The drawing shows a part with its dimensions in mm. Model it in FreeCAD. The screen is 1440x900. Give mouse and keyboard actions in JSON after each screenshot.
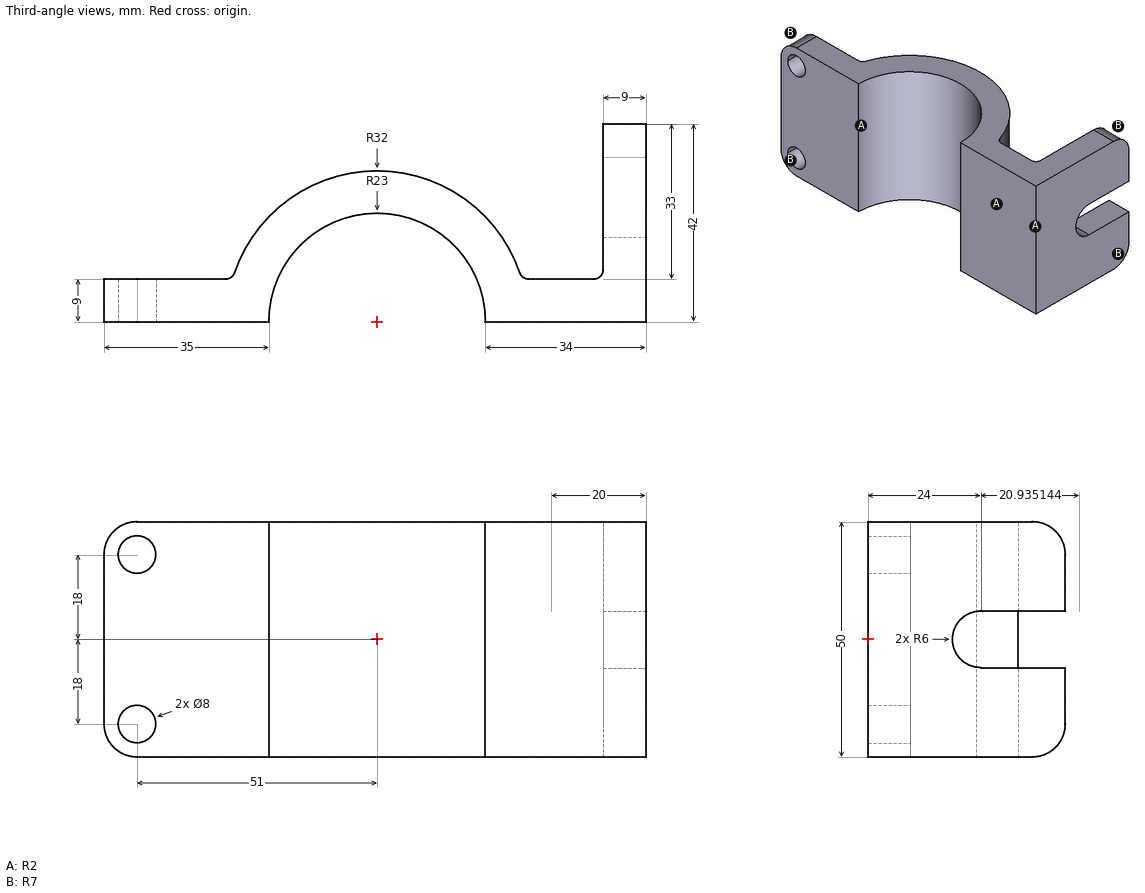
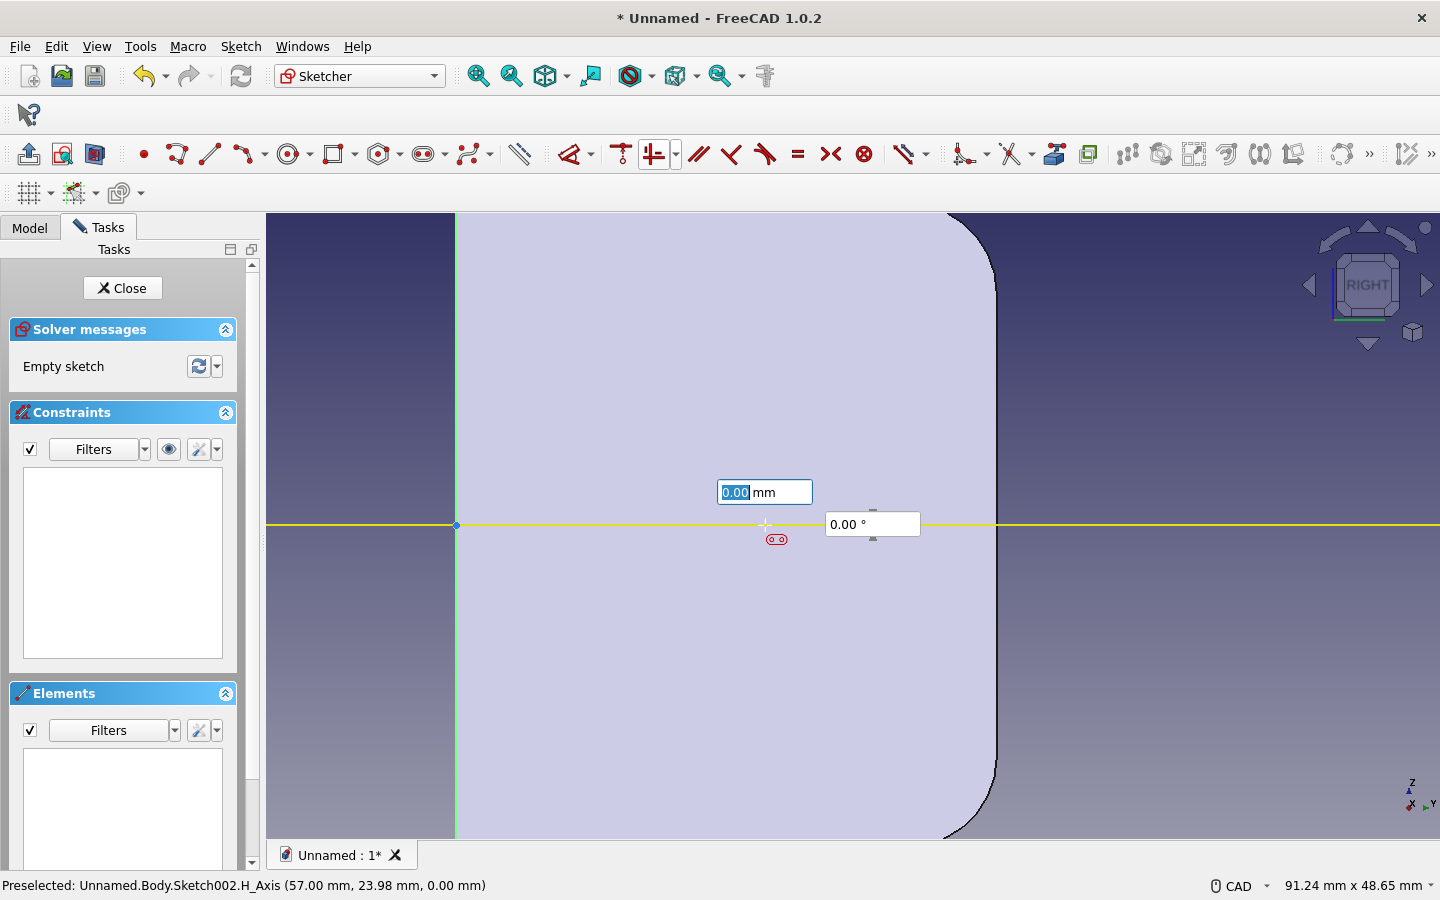
{"action": "left_click", "coordinate": [1035, 516]}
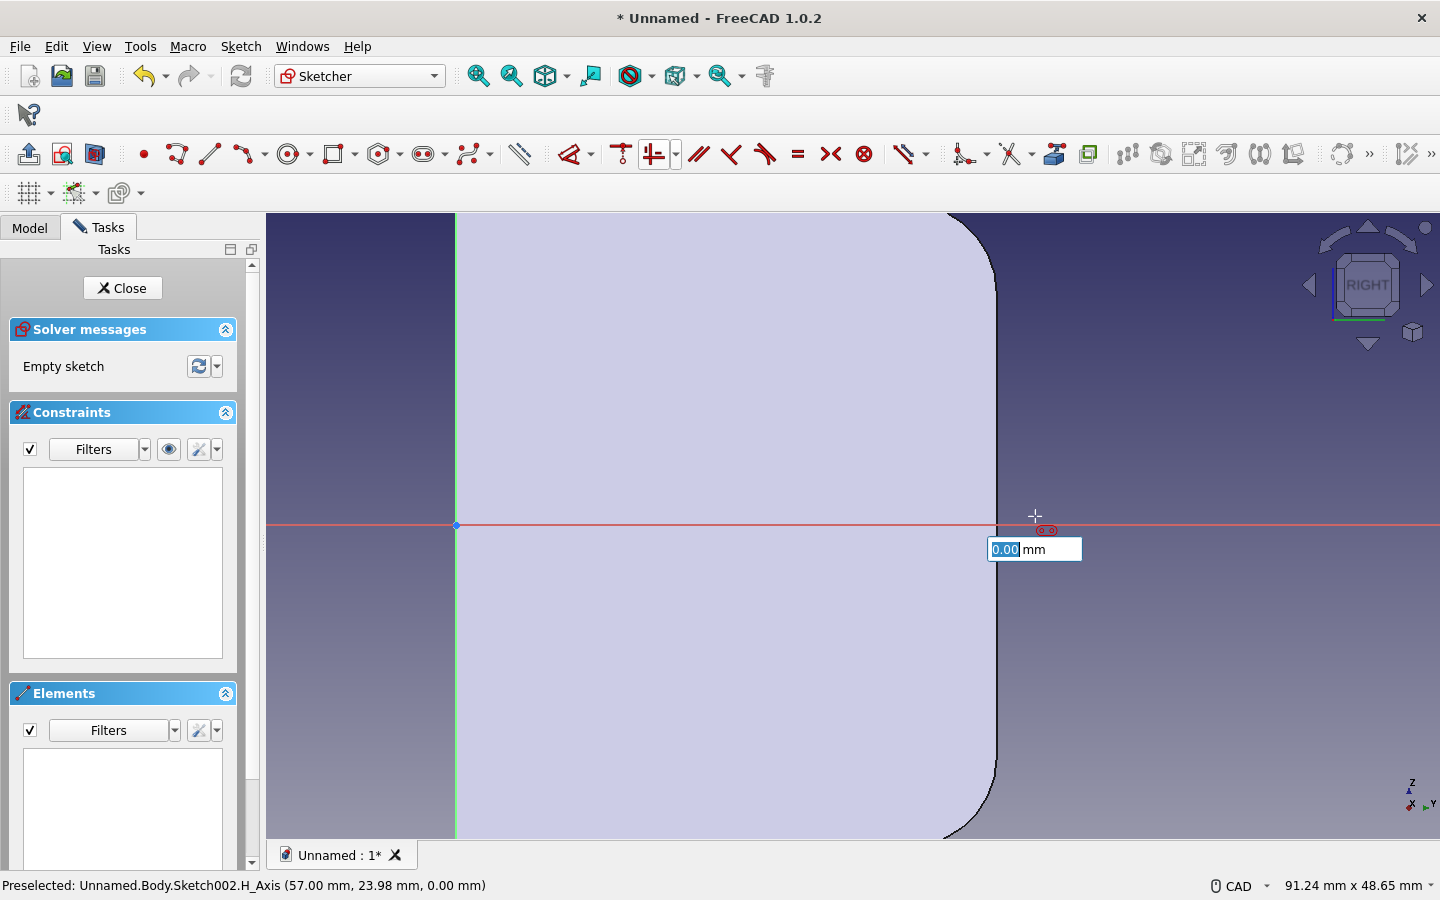
{"action": "left_click", "coordinate": [900, 448]}
{"action": "key", "text": "Escape"}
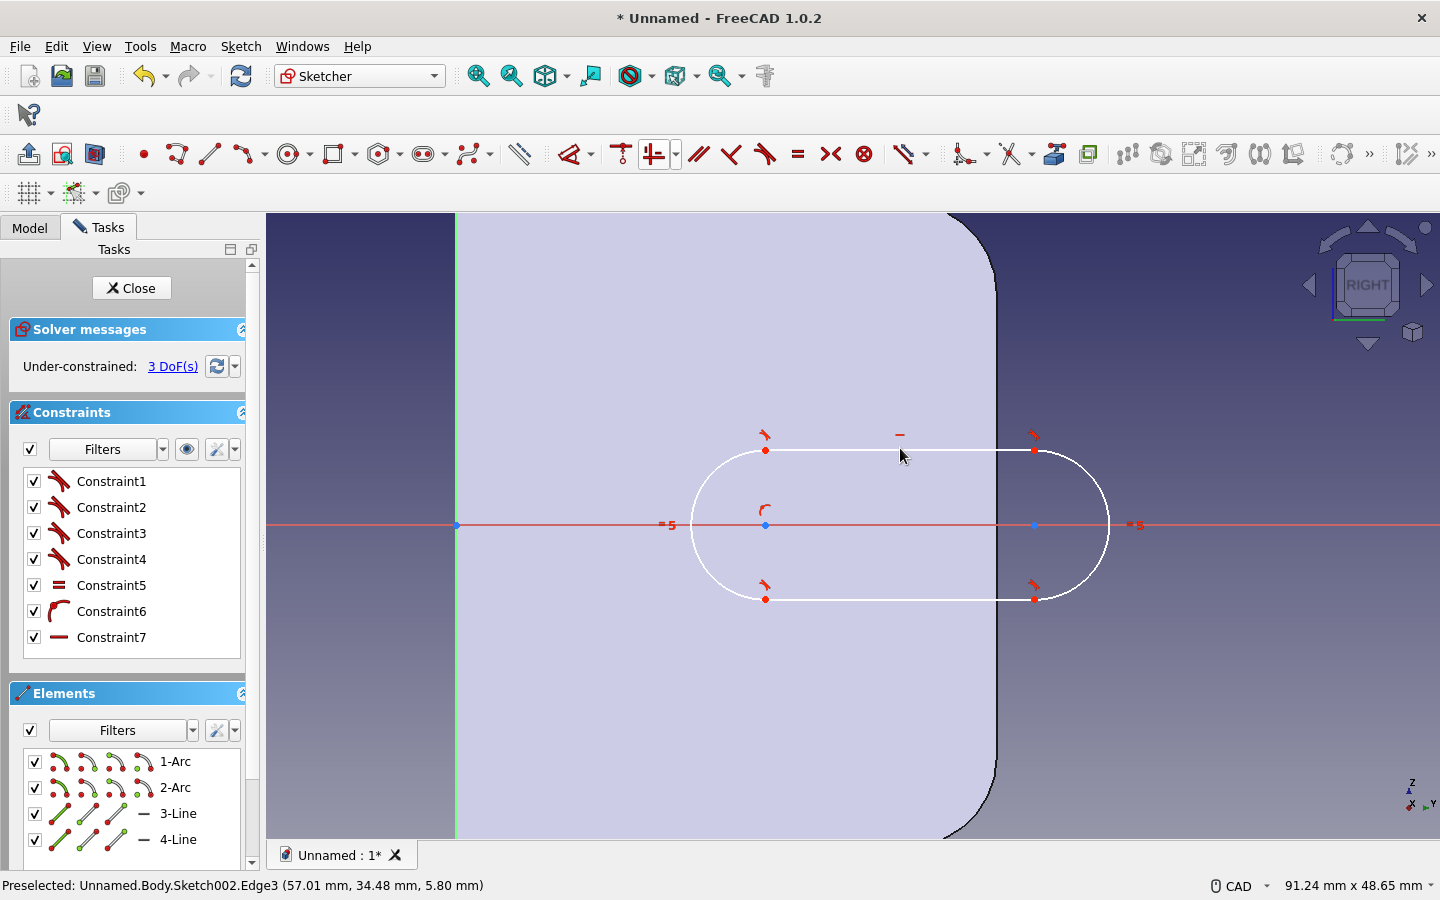
{"action": "left_click", "coordinate": [568, 154]}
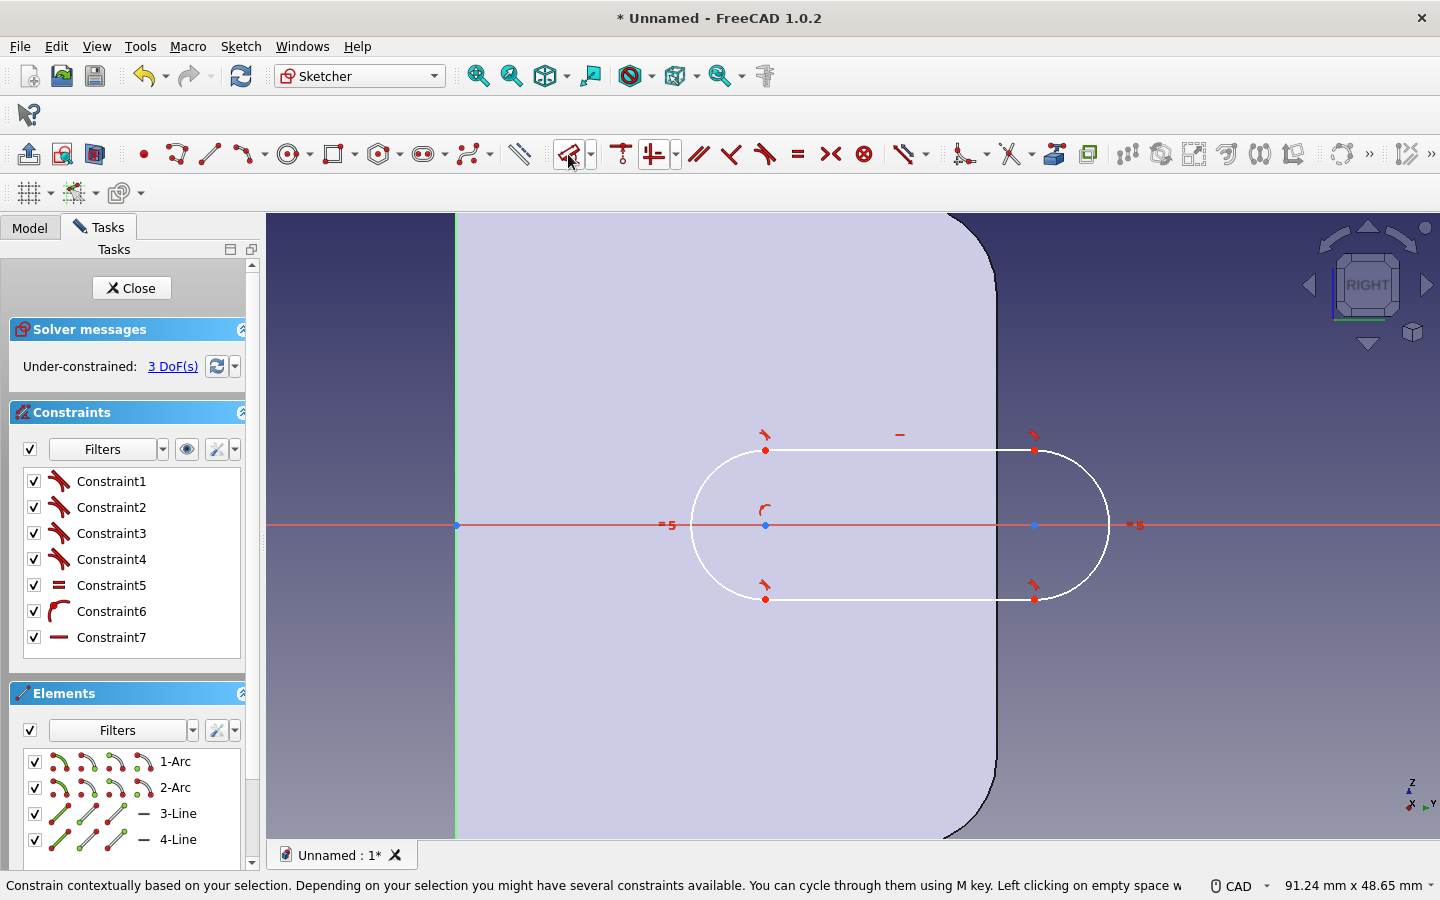
{"action": "left_click", "coordinate": [706, 481]}
{"action": "left_click", "coordinate": [680, 462]}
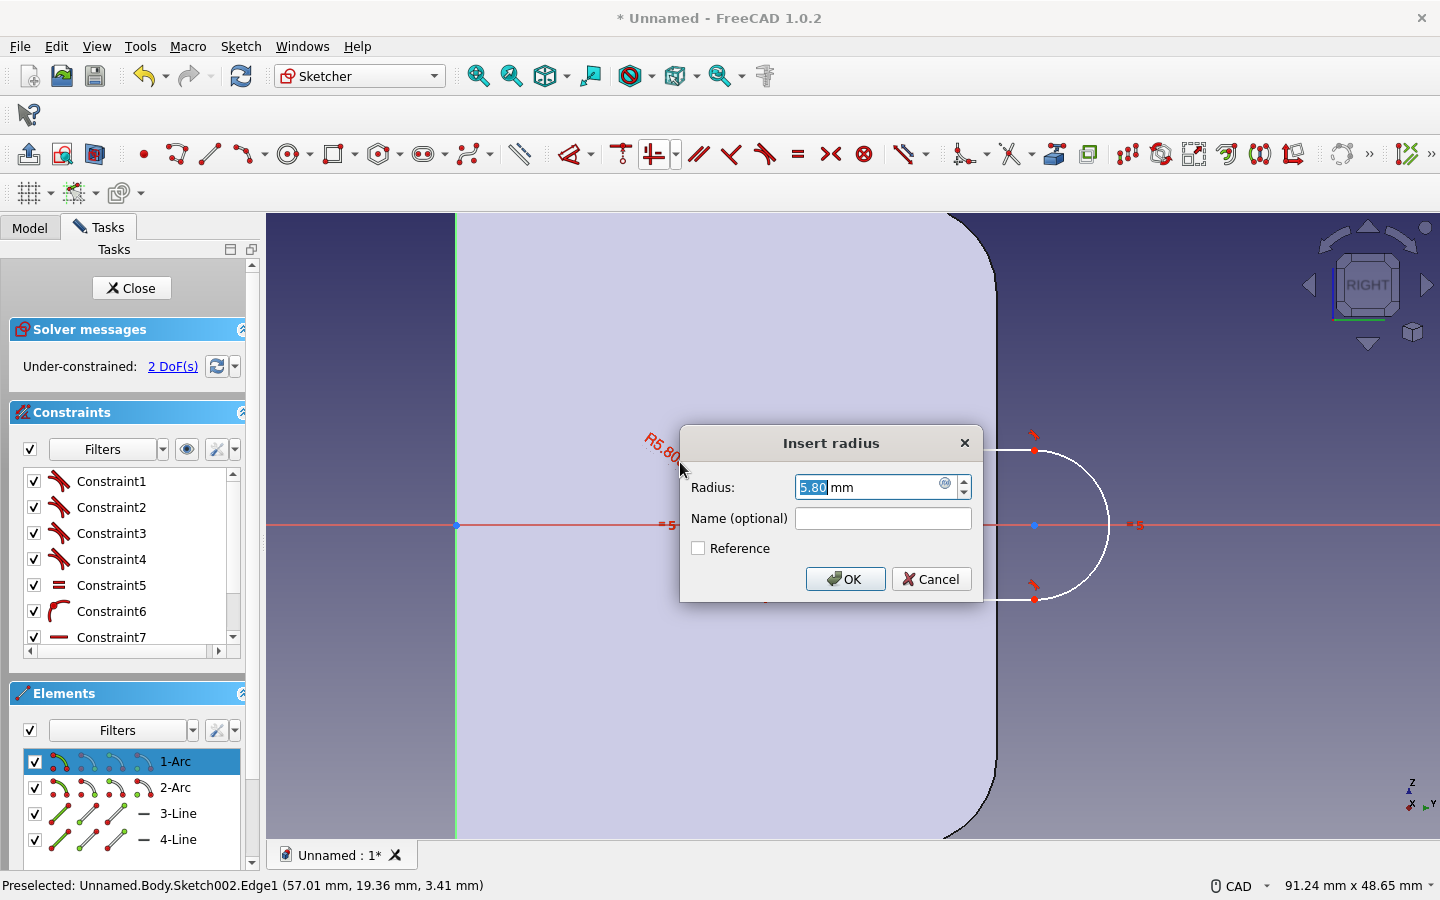
{"action": "type", "text": "6"}
{"action": "key", "text": "Return"}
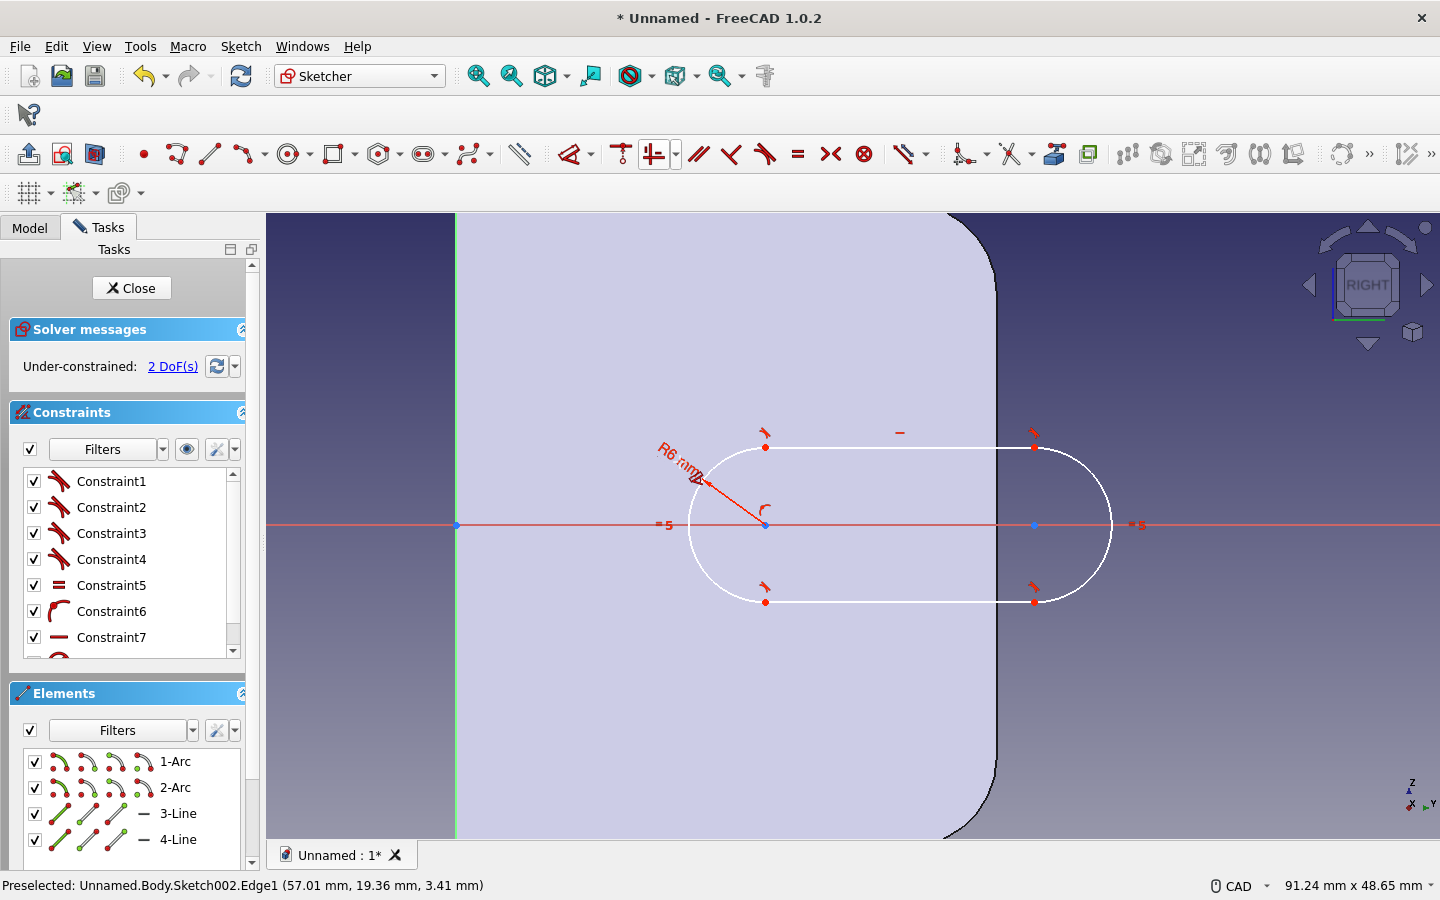
{"action": "left_click", "coordinate": [766, 448]}
{"action": "left_click", "coordinate": [611, 414]}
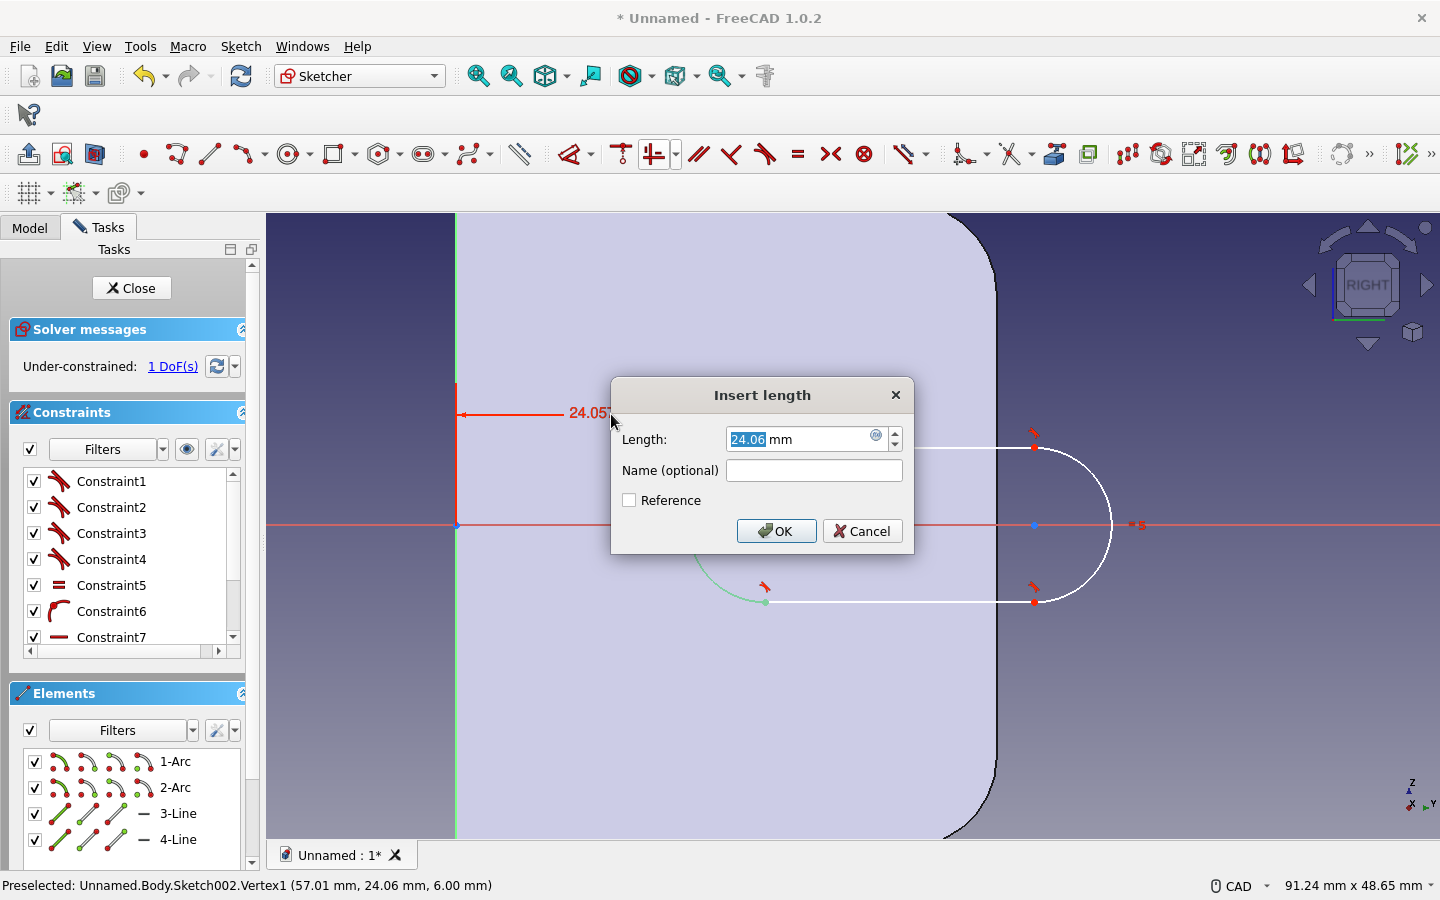
{"action": "type", "text": "24"}
{"action": "key", "text": "Return"}